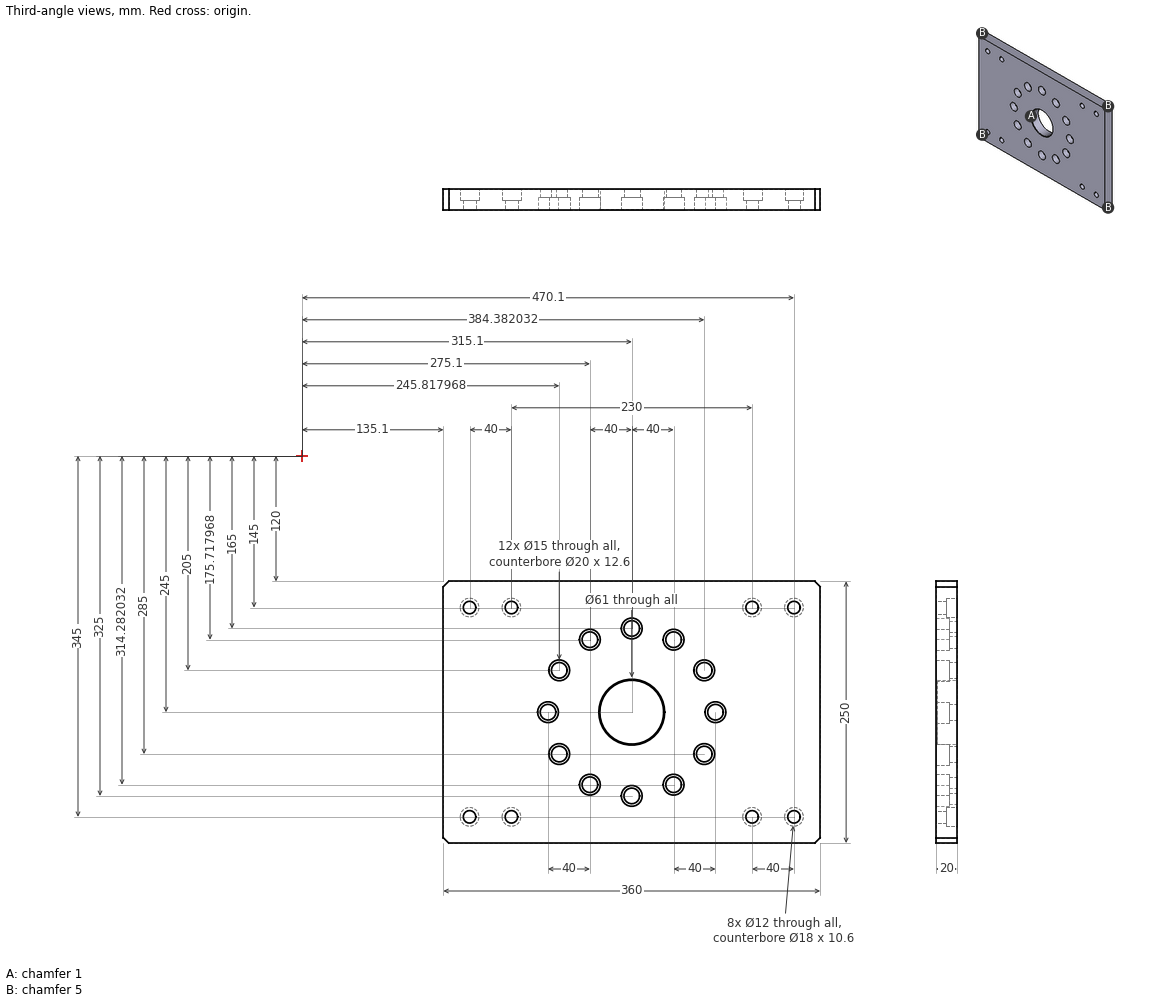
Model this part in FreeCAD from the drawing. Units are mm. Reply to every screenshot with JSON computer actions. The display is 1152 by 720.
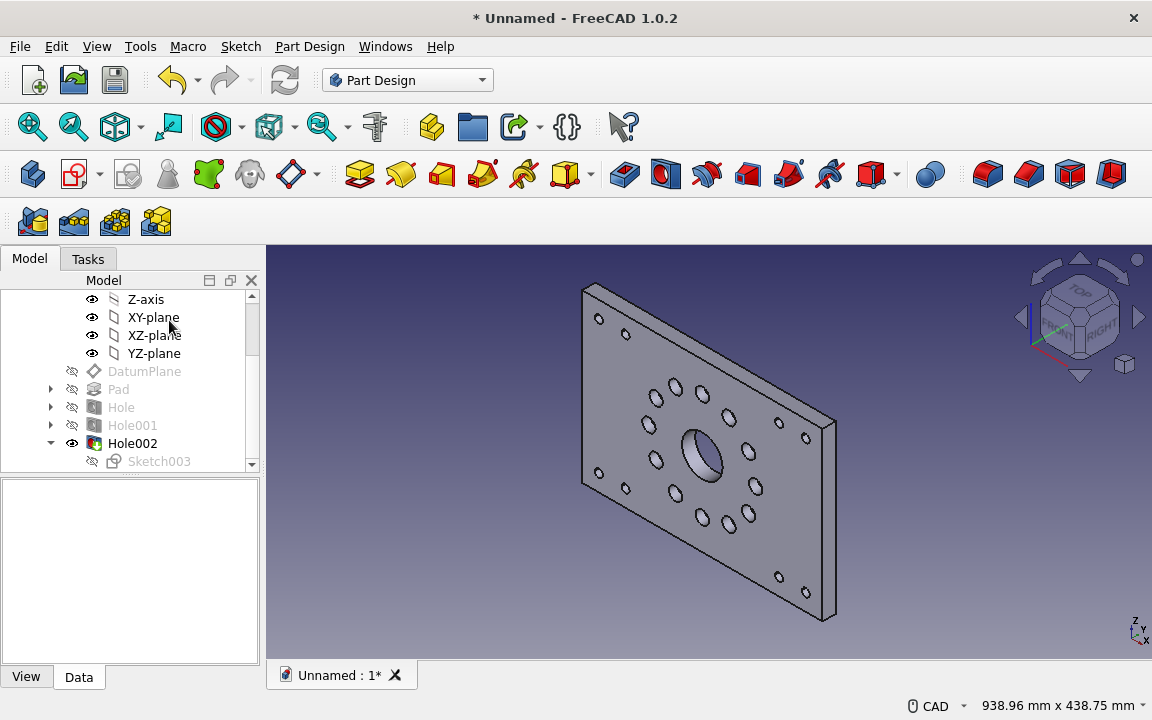
{"action": "left_click", "coordinate": [682, 443]}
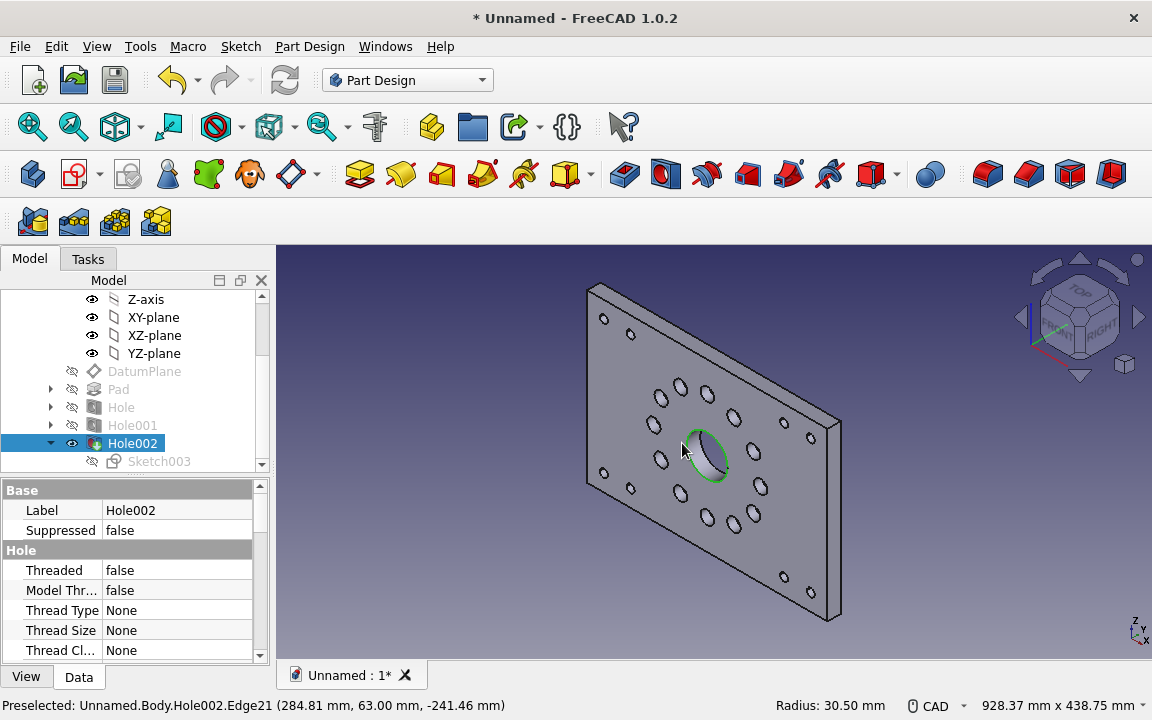
{"action": "left_click", "coordinate": [1029, 174]}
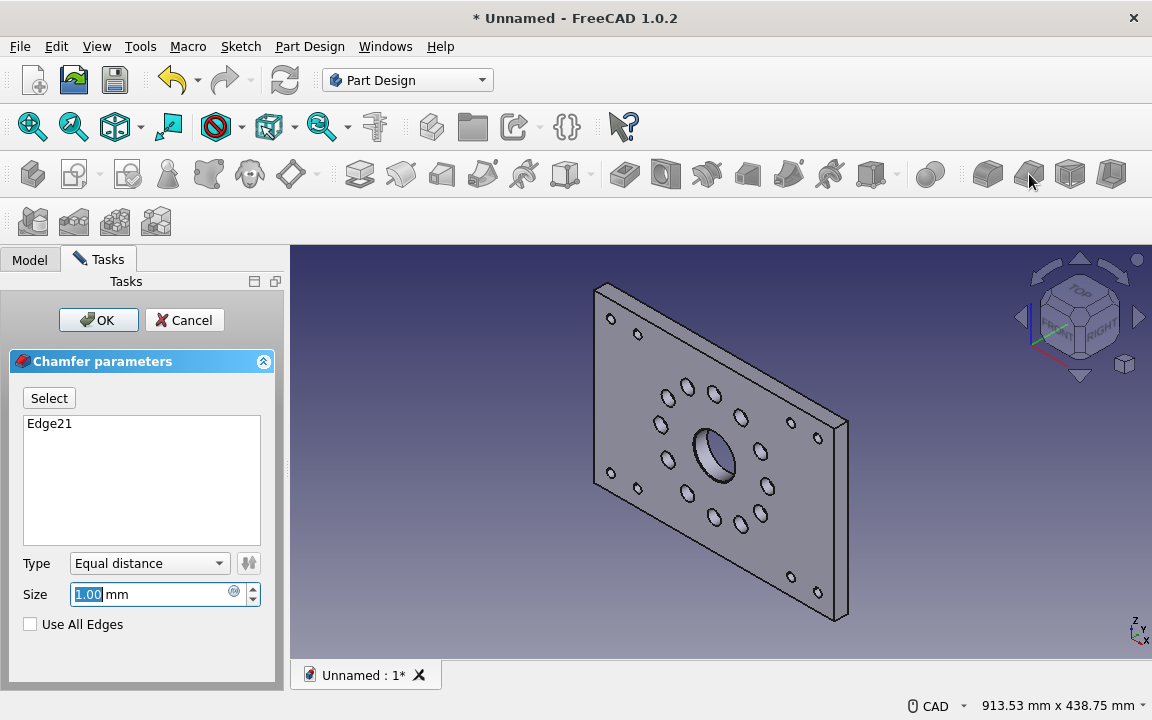
{"action": "type", "text": "1"}
{"action": "key", "text": "Tab"}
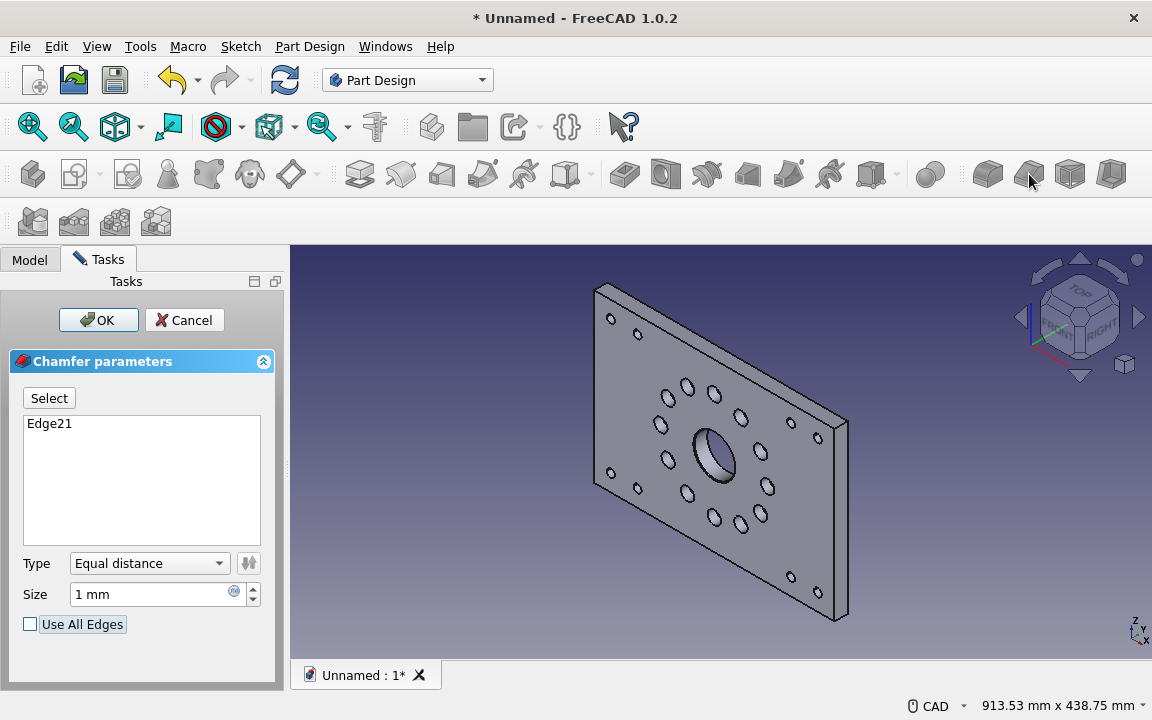
{"action": "left_click", "coordinate": [99, 320]}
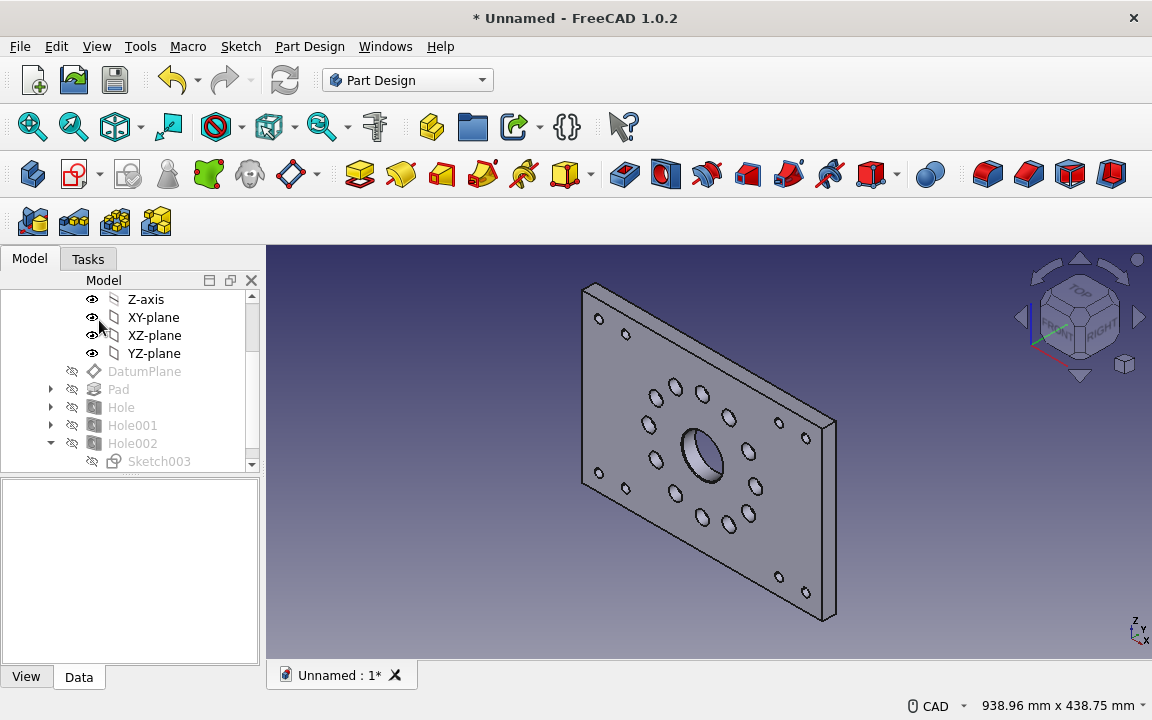
{"action": "left_click", "coordinate": [829, 424]}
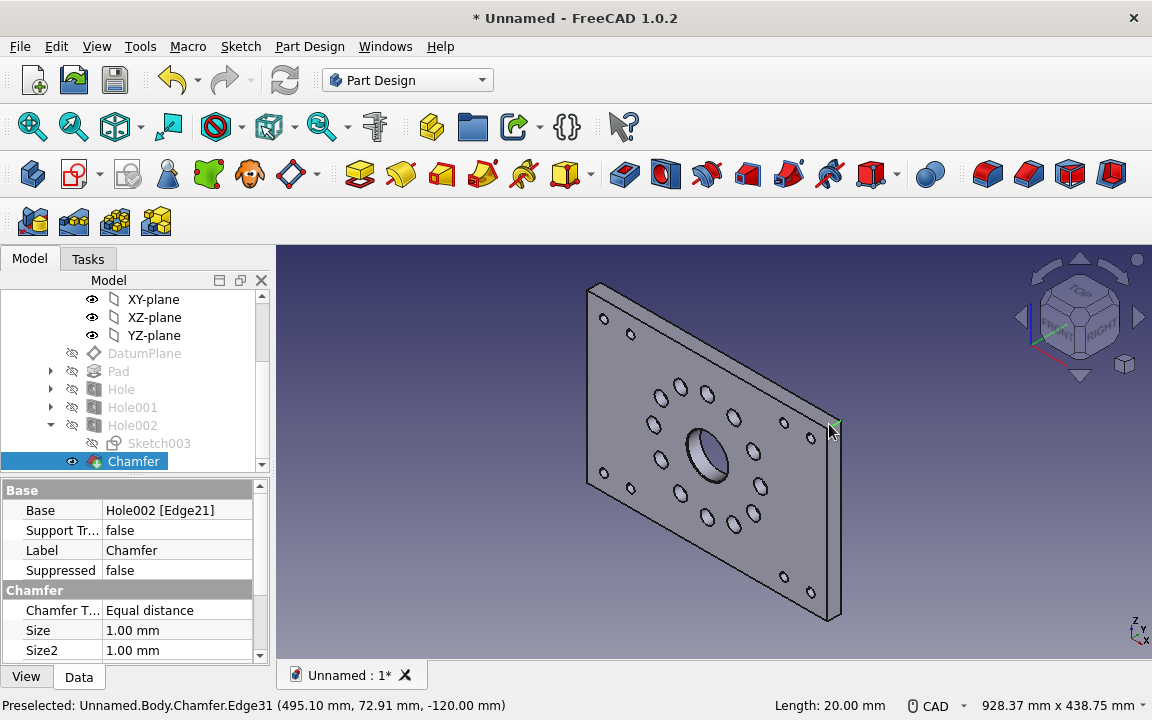
{"action": "scroll", "coordinate": [834, 617], "scroll_direction": "up", "scroll_amount": 4}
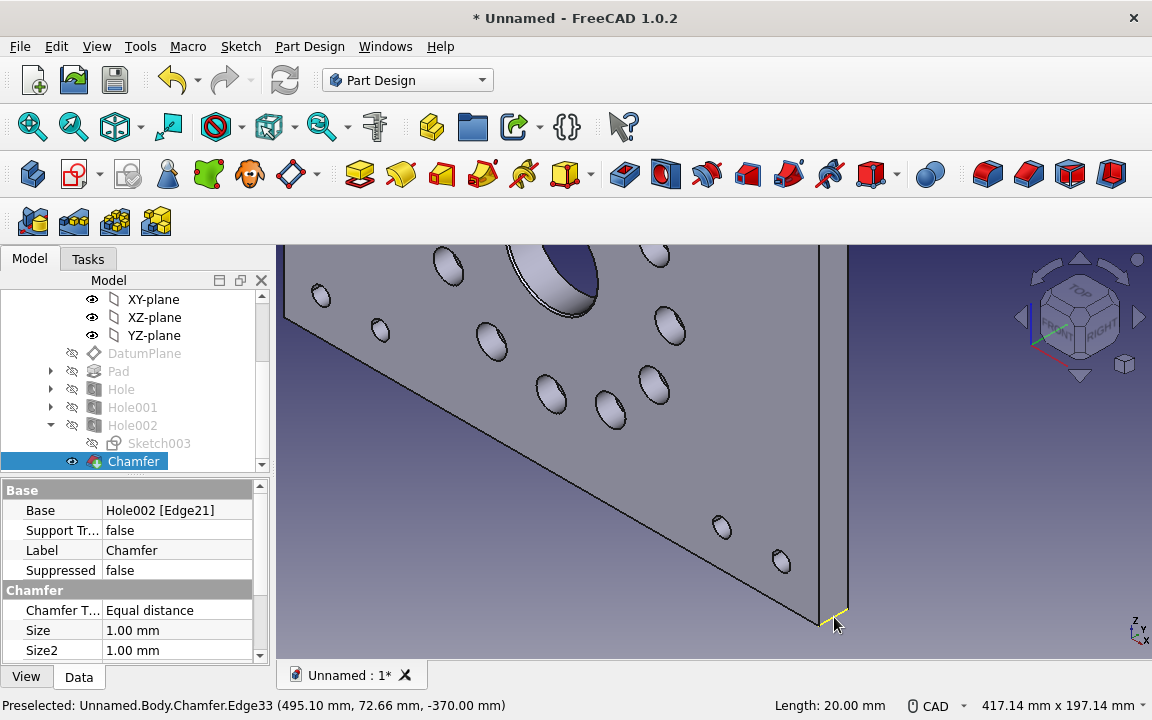
{"action": "left_click", "coordinate": [33, 128]}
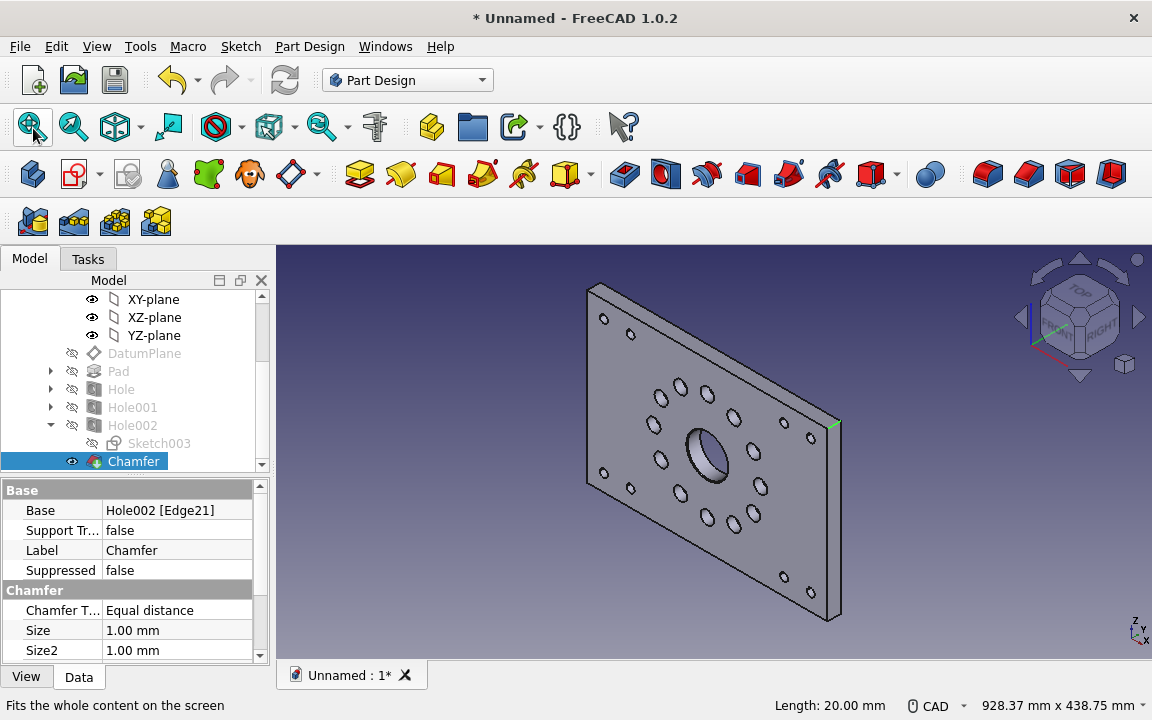
{"action": "key", "text": "2"}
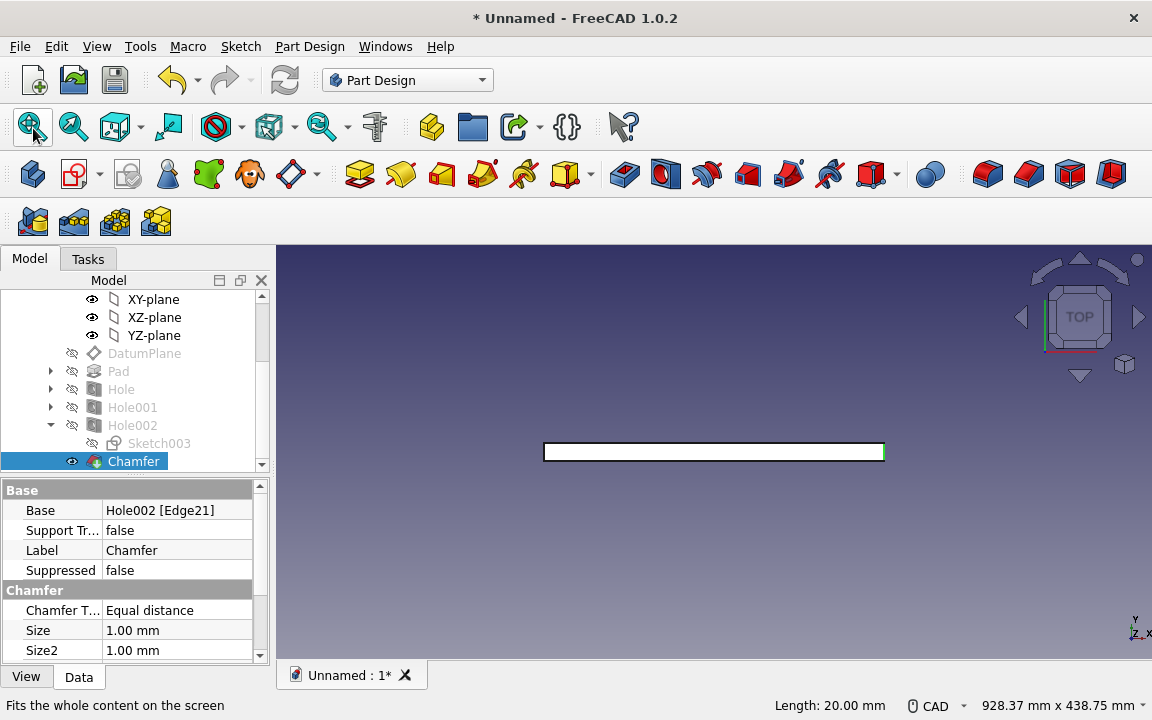
{"action": "left_click", "coordinate": [33, 128]}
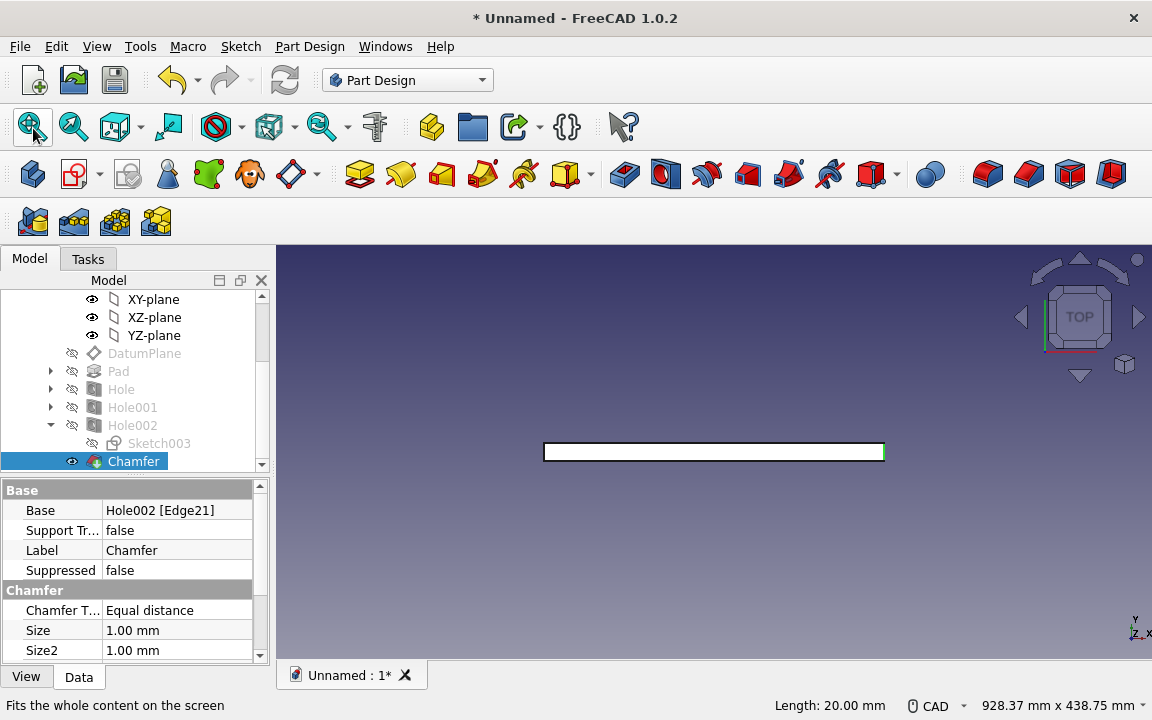
{"action": "left_click", "coordinate": [544, 451], "text": "ctrl"}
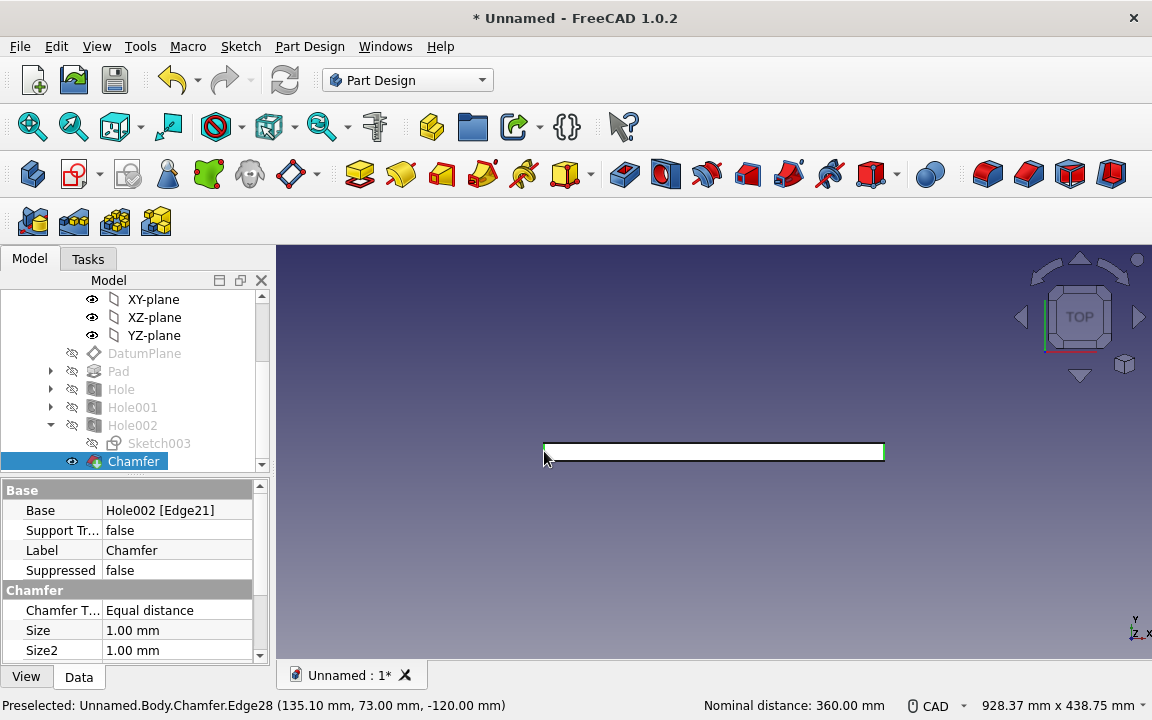
{"action": "scroll", "coordinate": [884, 451], "scroll_direction": "up", "scroll_amount": 4}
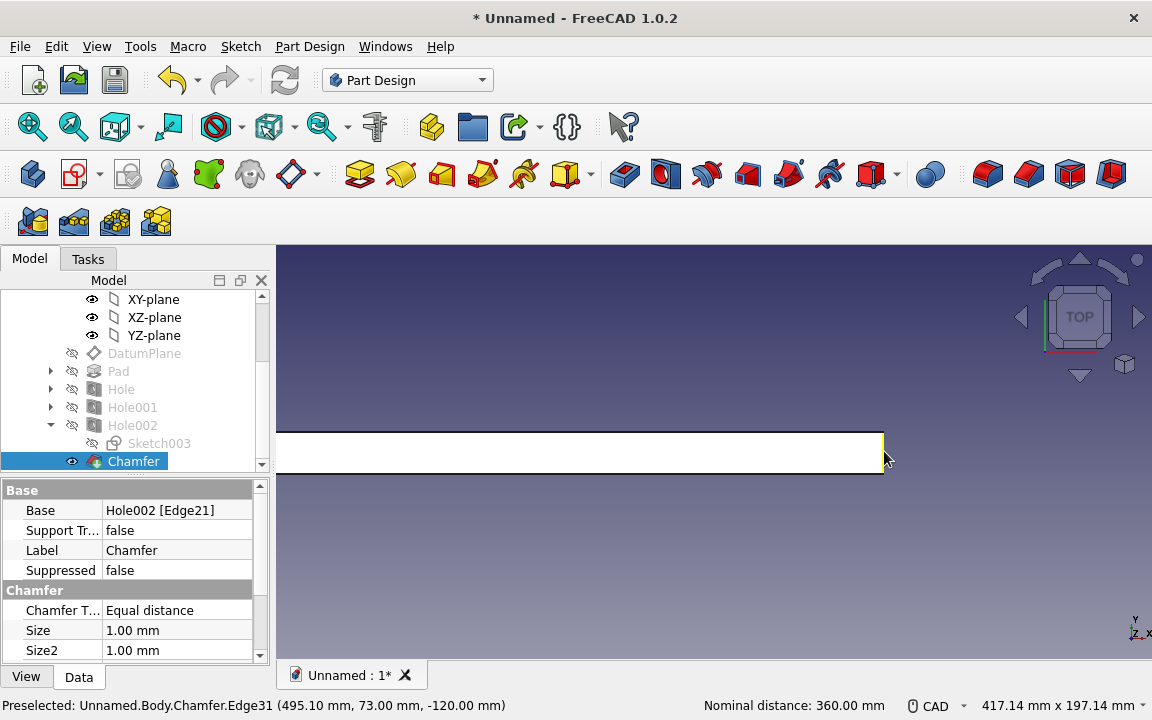
{"action": "left_click", "coordinate": [33, 128]}